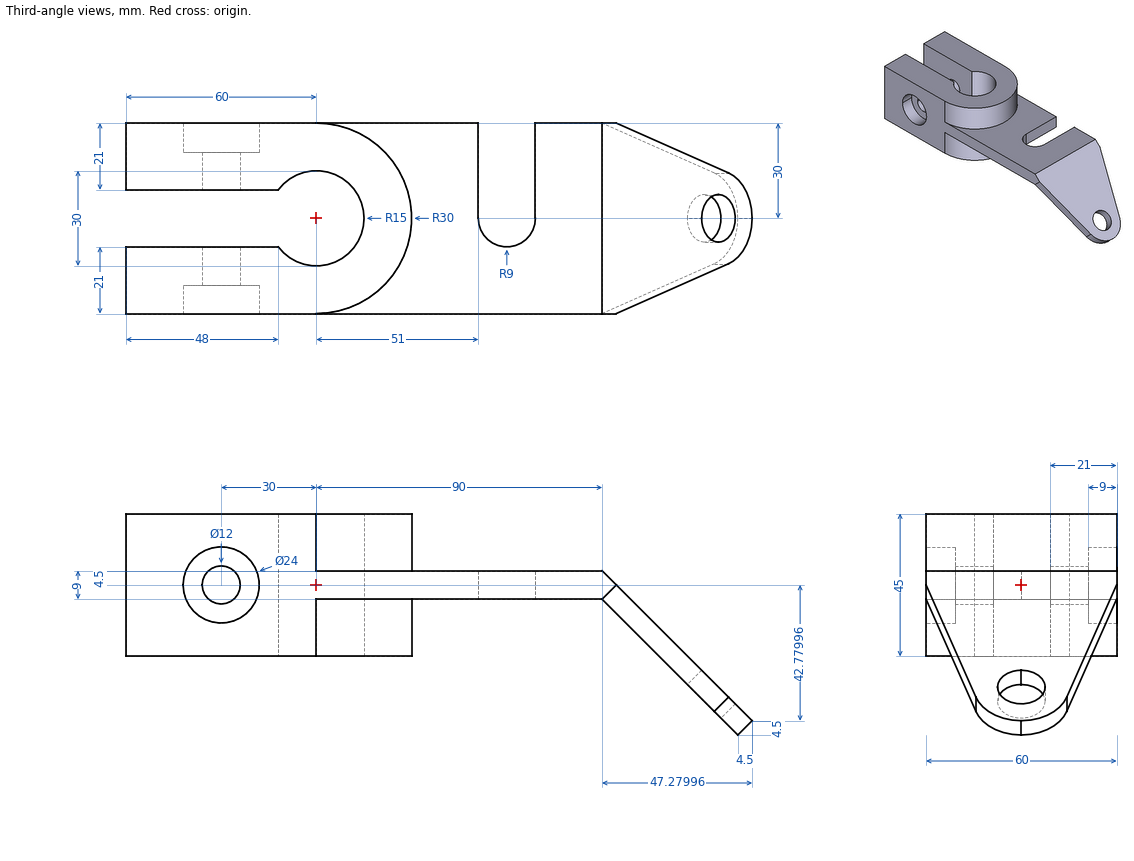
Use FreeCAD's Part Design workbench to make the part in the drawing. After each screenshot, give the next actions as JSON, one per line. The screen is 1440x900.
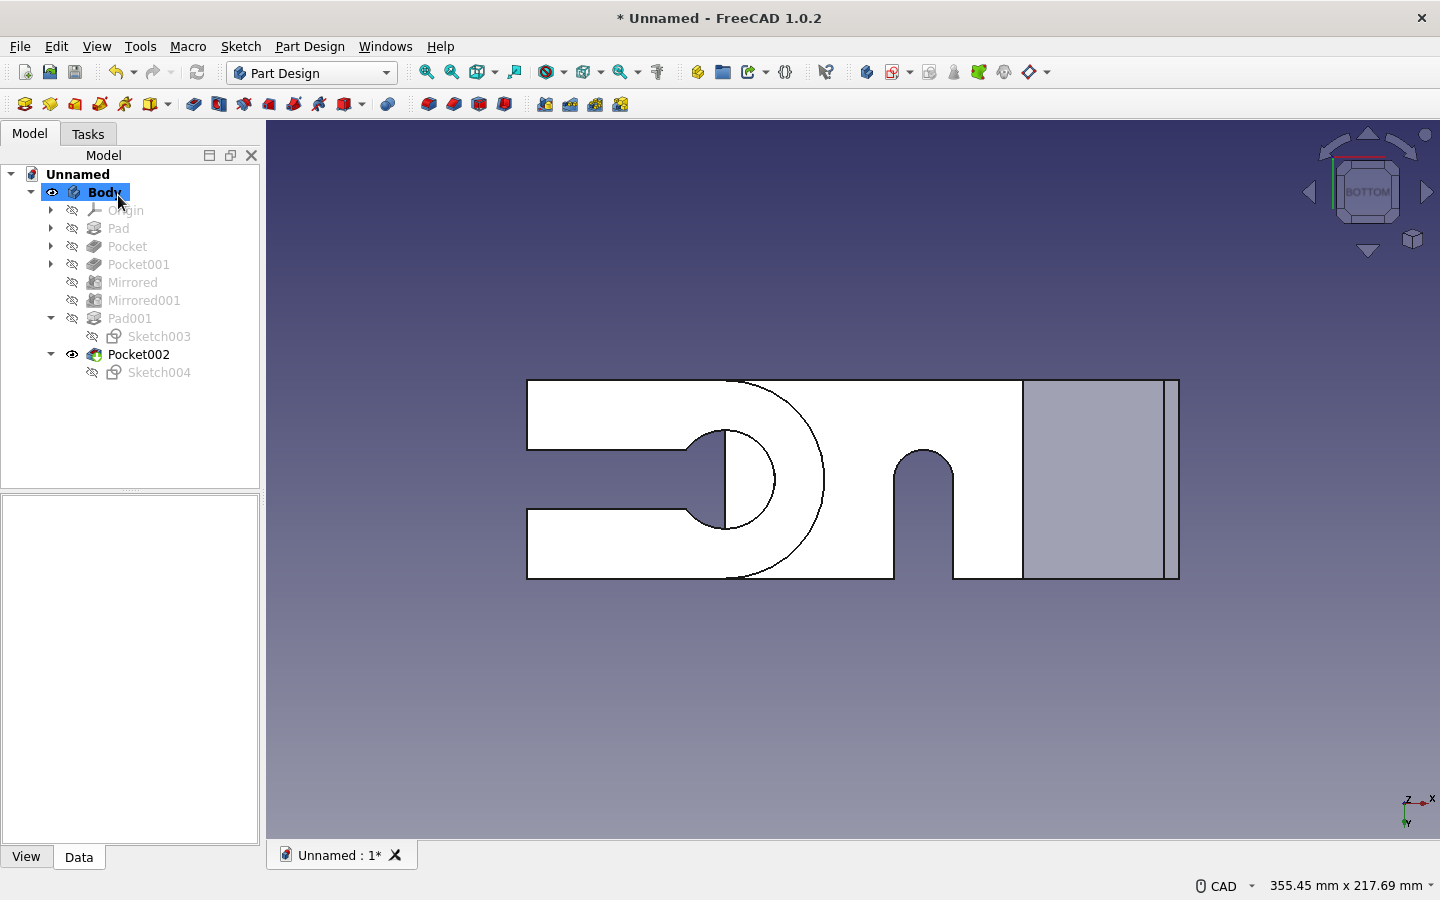
{"action": "left_click", "coordinate": [1093, 479]}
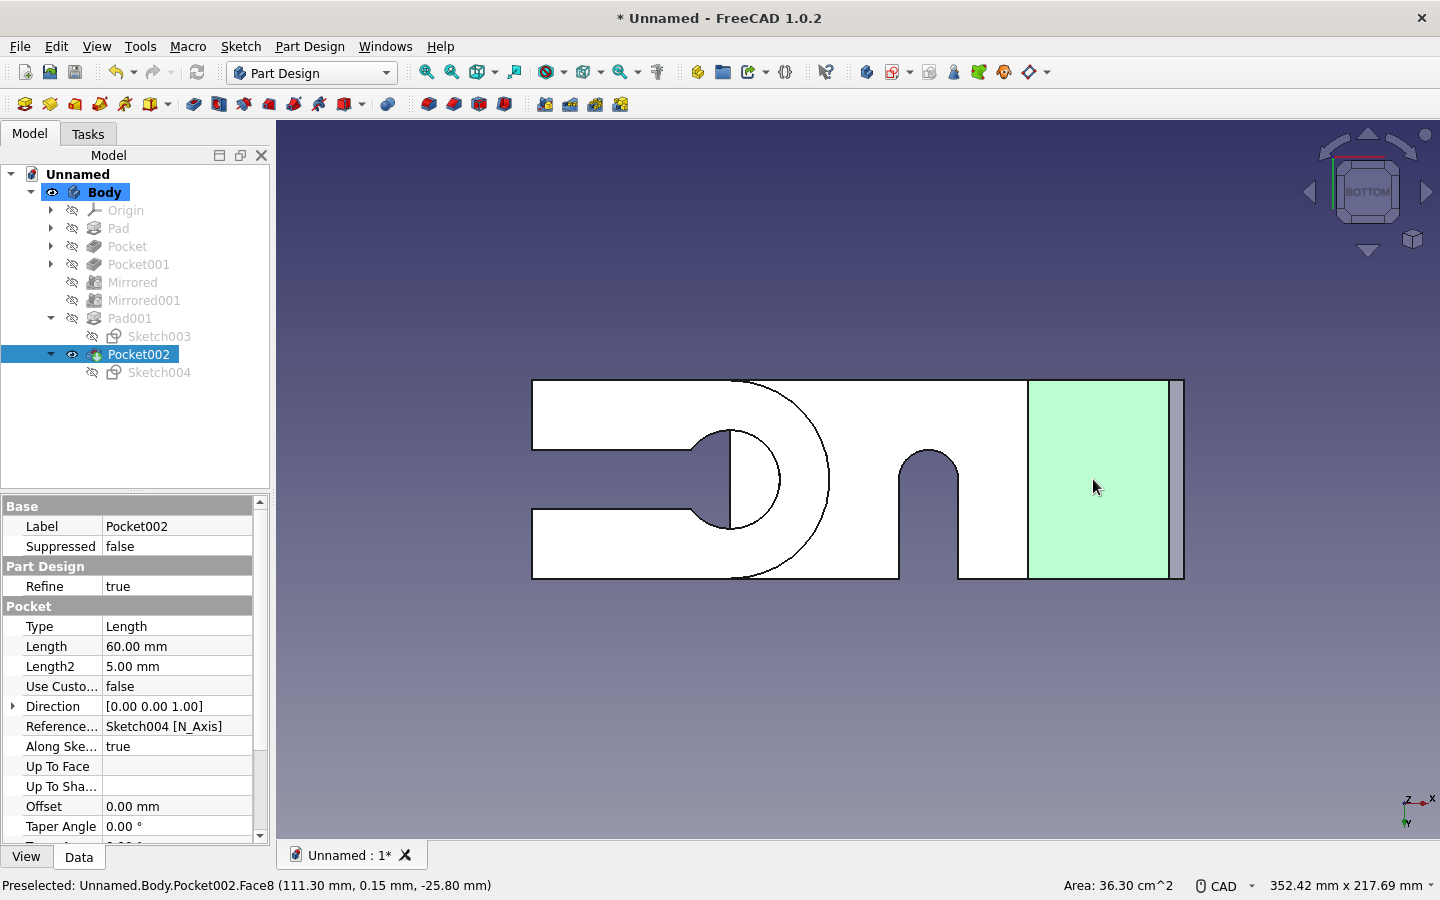
{"action": "left_click", "coordinate": [892, 72]}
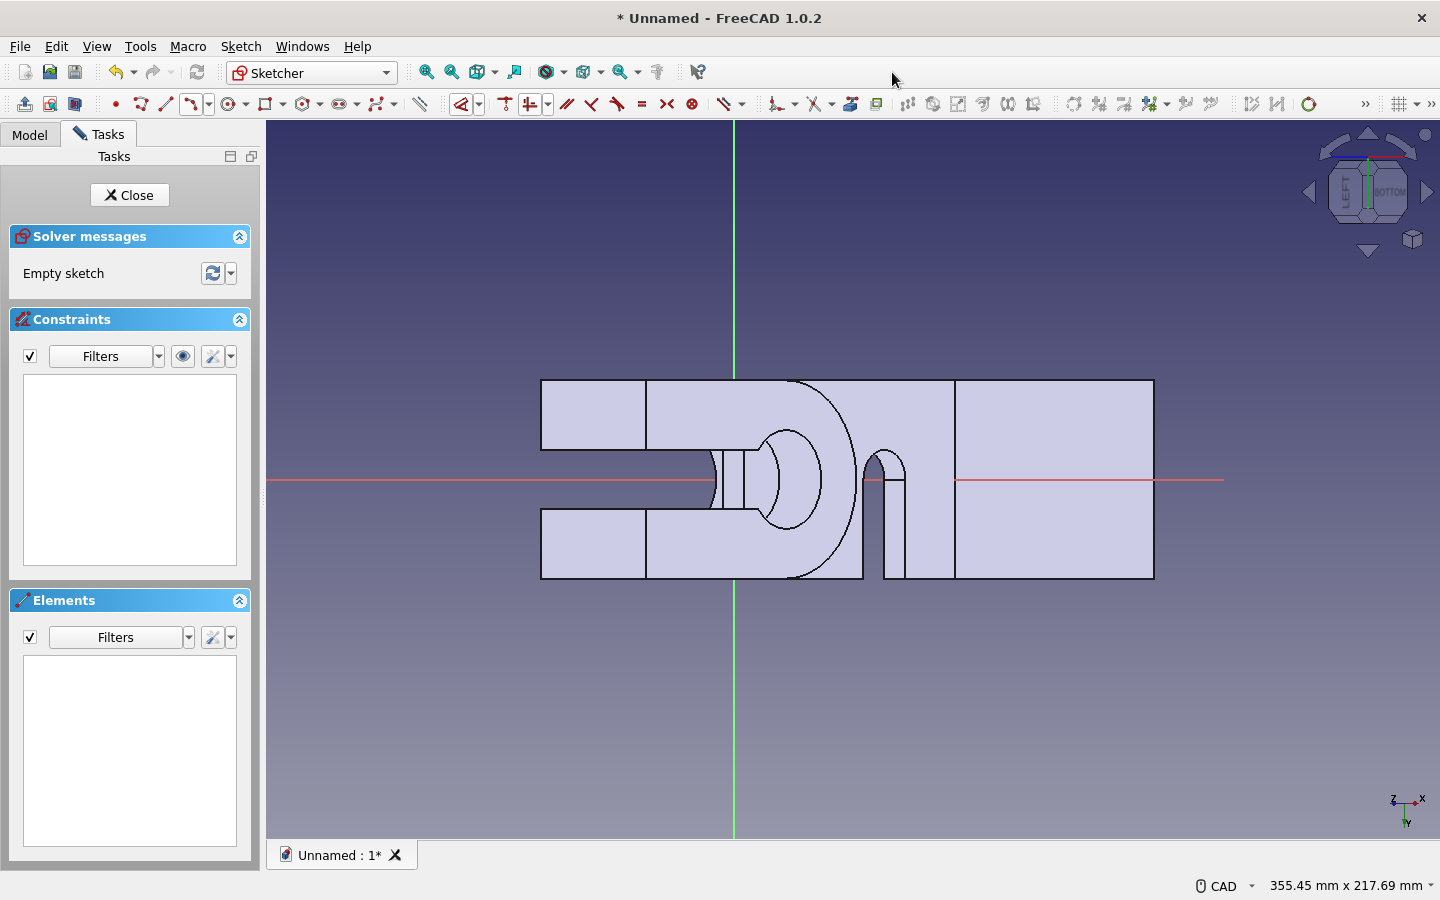
{"action": "scroll", "coordinate": [1269, 480], "scroll_direction": "up", "scroll_amount": 2}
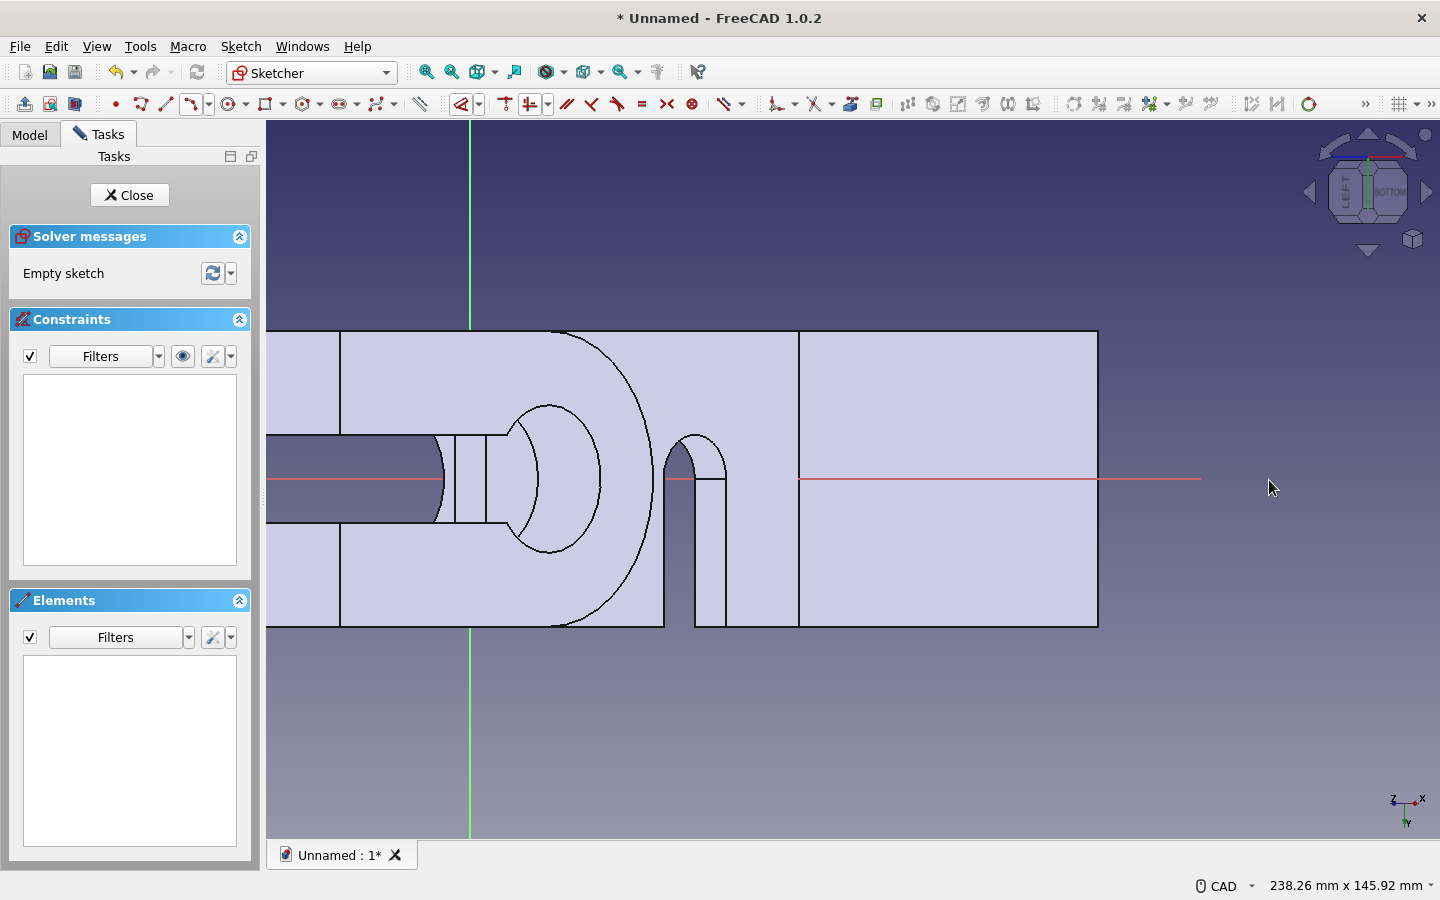
{"action": "left_click", "coordinate": [141, 104]}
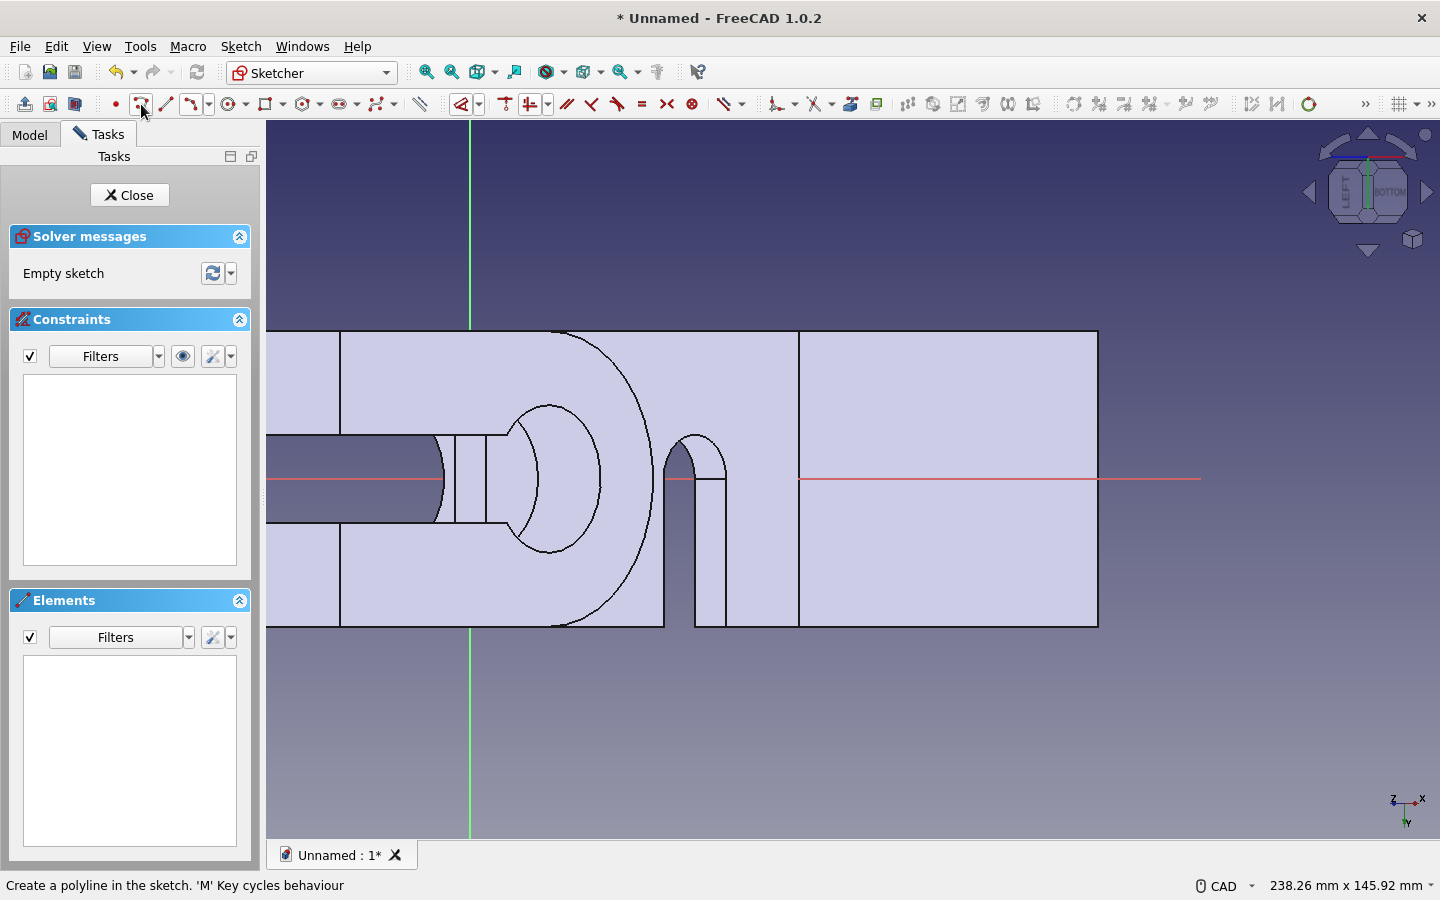
{"action": "left_click", "coordinate": [1046, 550]}
{"action": "left_click", "coordinate": [799, 627]}
{"action": "left_click", "coordinate": [1098, 627]}
{"action": "left_click", "coordinate": [1098, 479]}
{"action": "right_click", "coordinate": [1098, 479]}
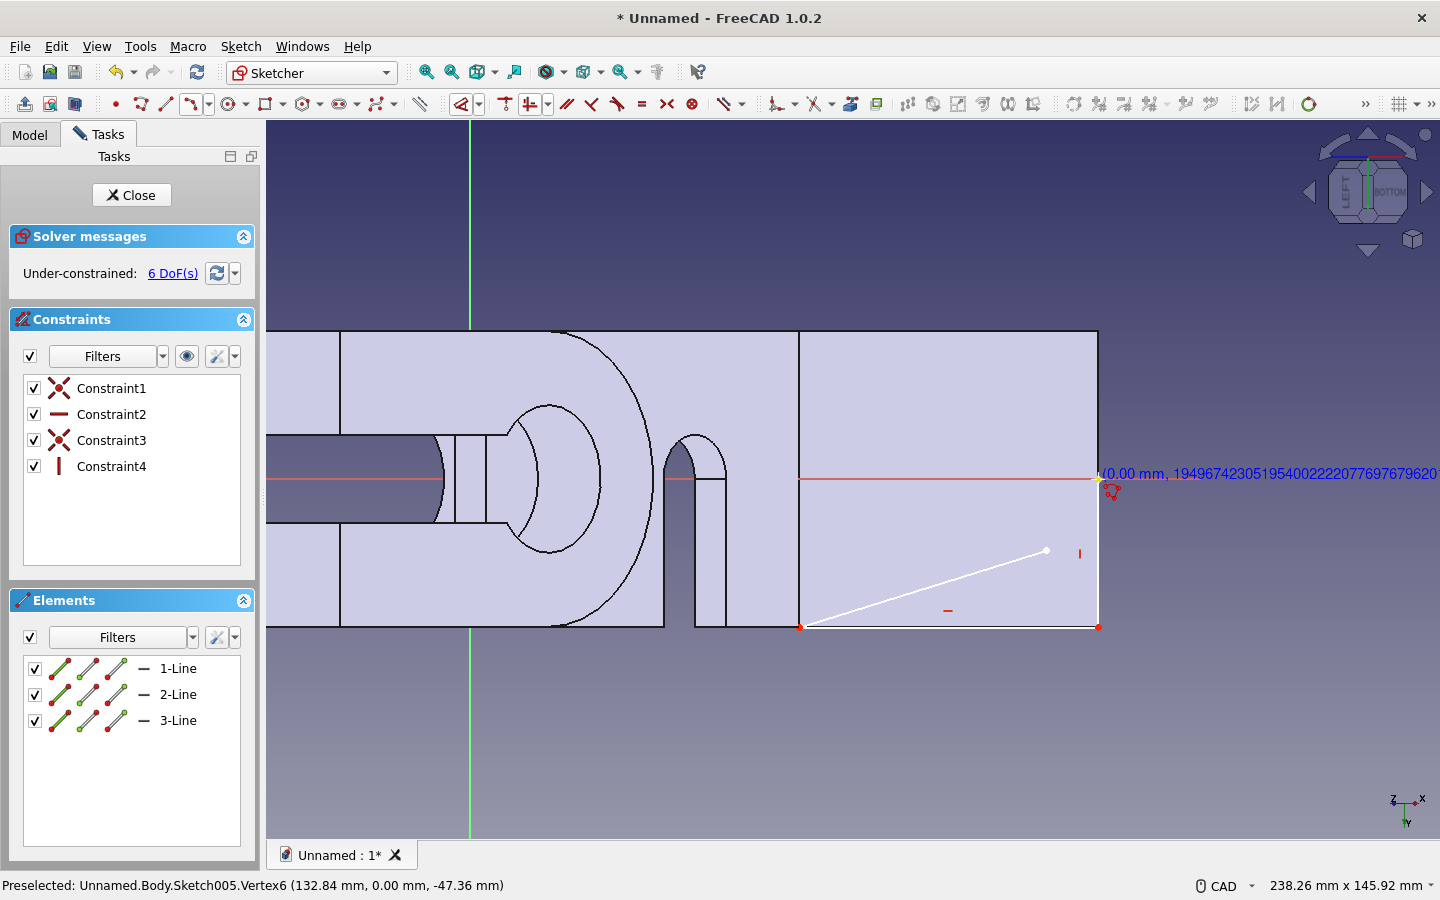
{"action": "left_click", "coordinate": [190, 104]}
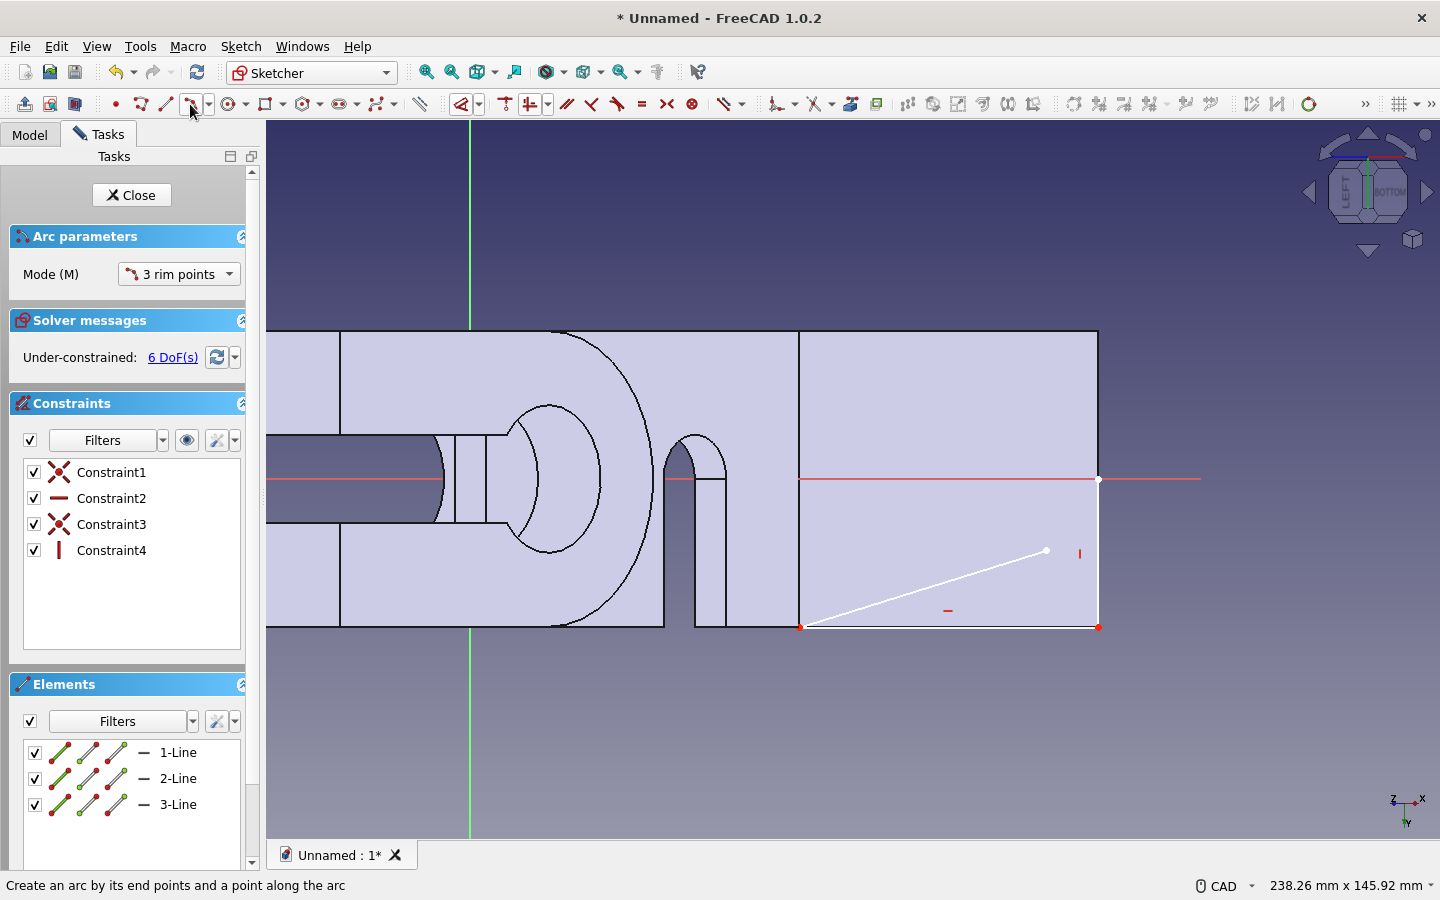
{"action": "left_click", "coordinate": [1098, 479]}
{"action": "left_click", "coordinate": [1046, 551]}
{"action": "left_click", "coordinate": [1083, 523]}